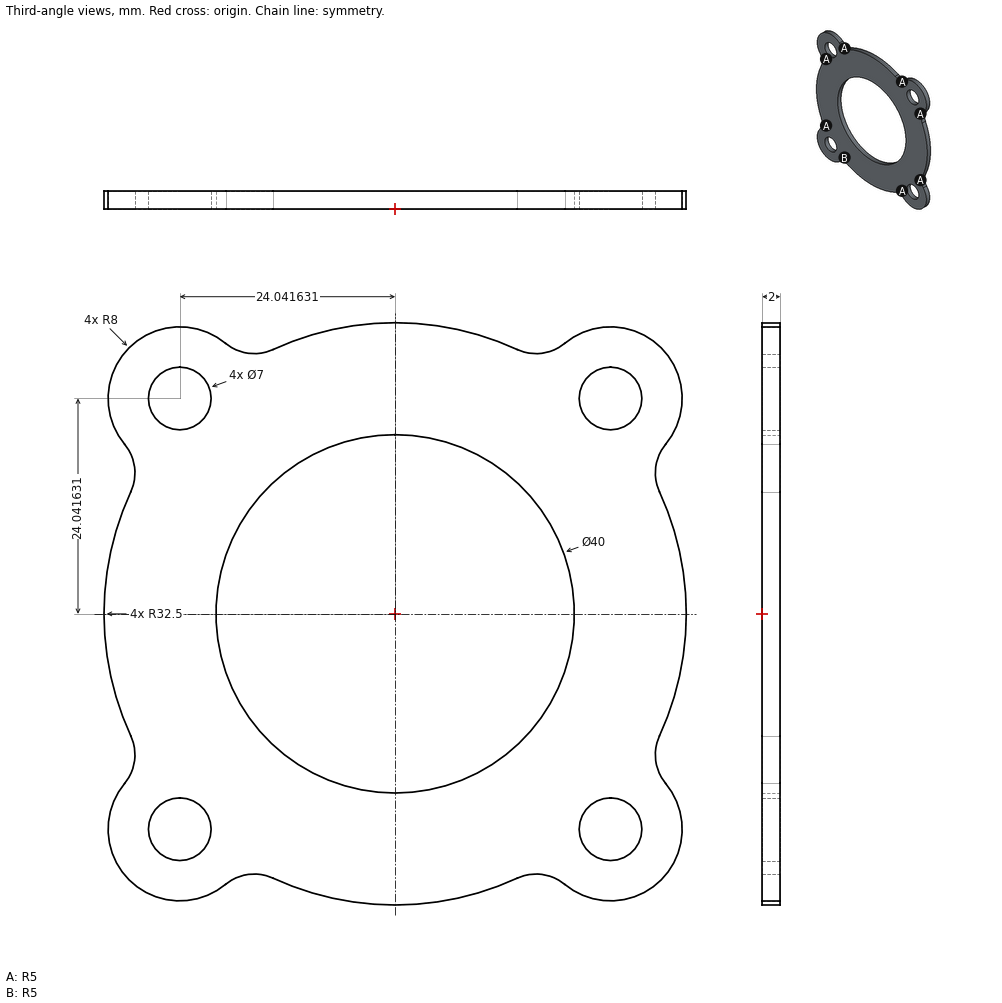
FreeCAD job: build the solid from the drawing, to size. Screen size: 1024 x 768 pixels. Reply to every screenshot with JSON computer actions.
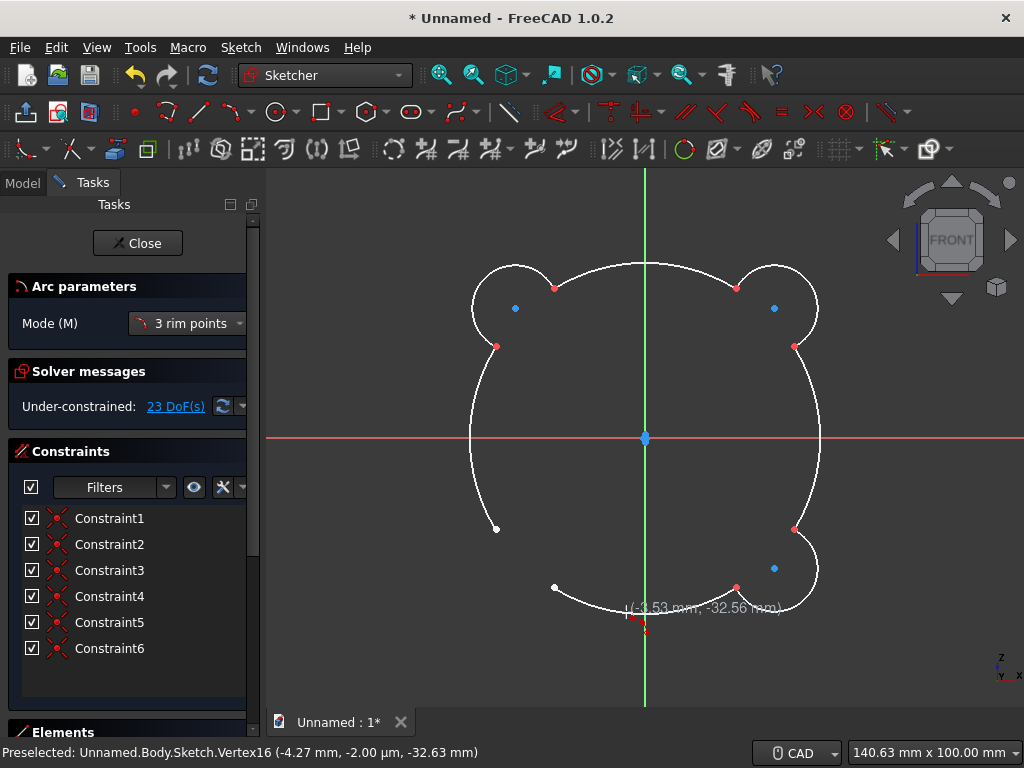
{"action": "left_click", "coordinate": [554, 588]}
{"action": "left_click", "coordinate": [496, 530]}
{"action": "left_click", "coordinate": [485, 598]}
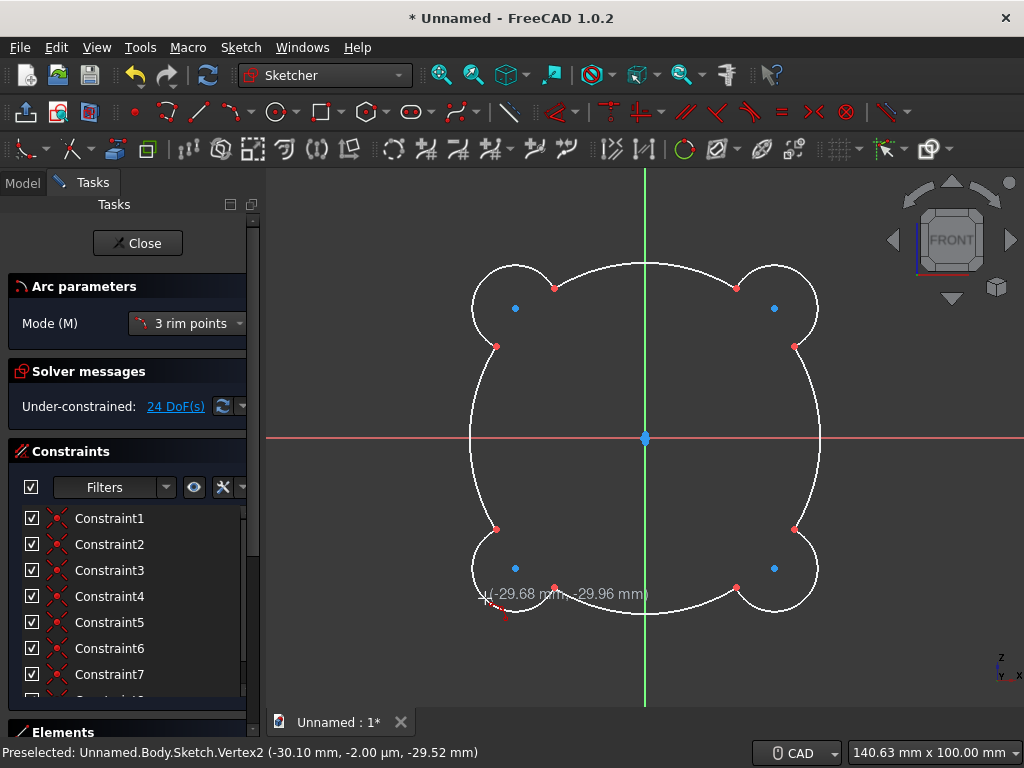
{"action": "left_click", "coordinate": [276, 112]}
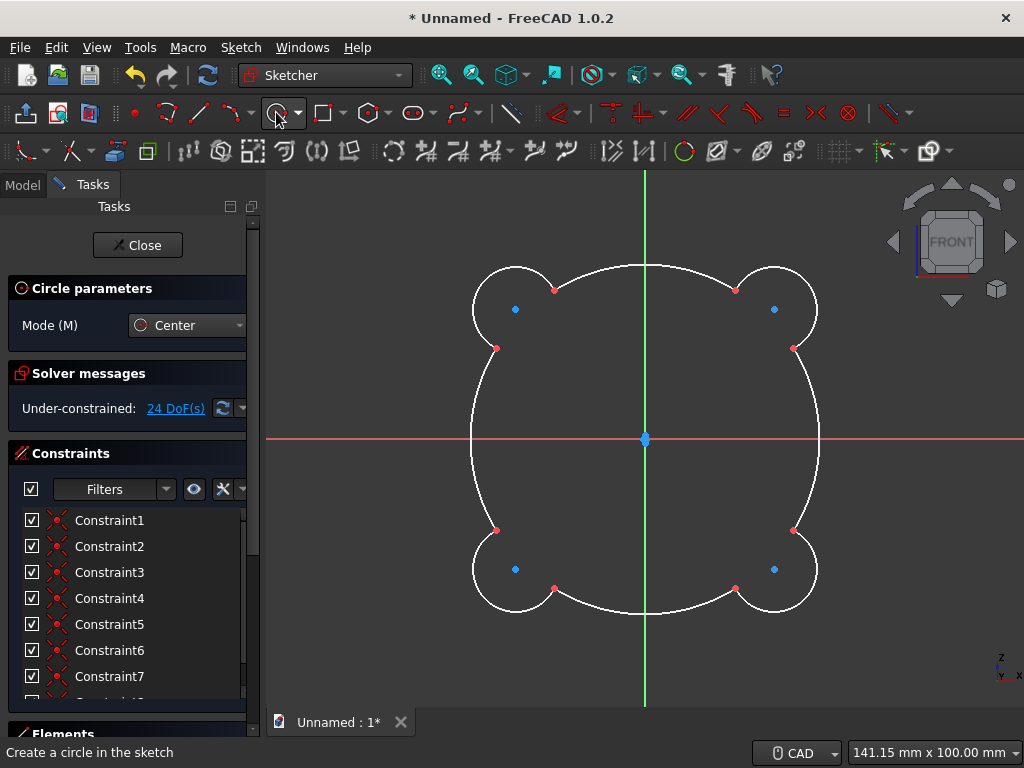
{"action": "left_click", "coordinate": [516, 309]}
{"action": "left_click", "coordinate": [529, 296]}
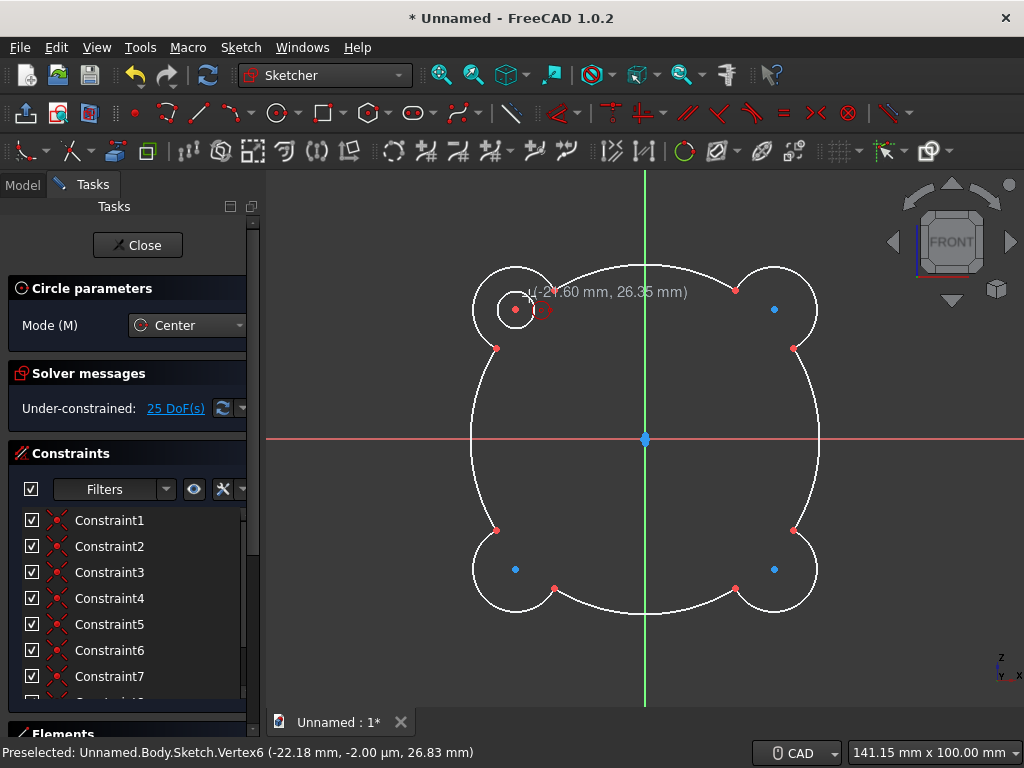
{"action": "left_click", "coordinate": [774, 309]}
{"action": "left_click", "coordinate": [787, 296]}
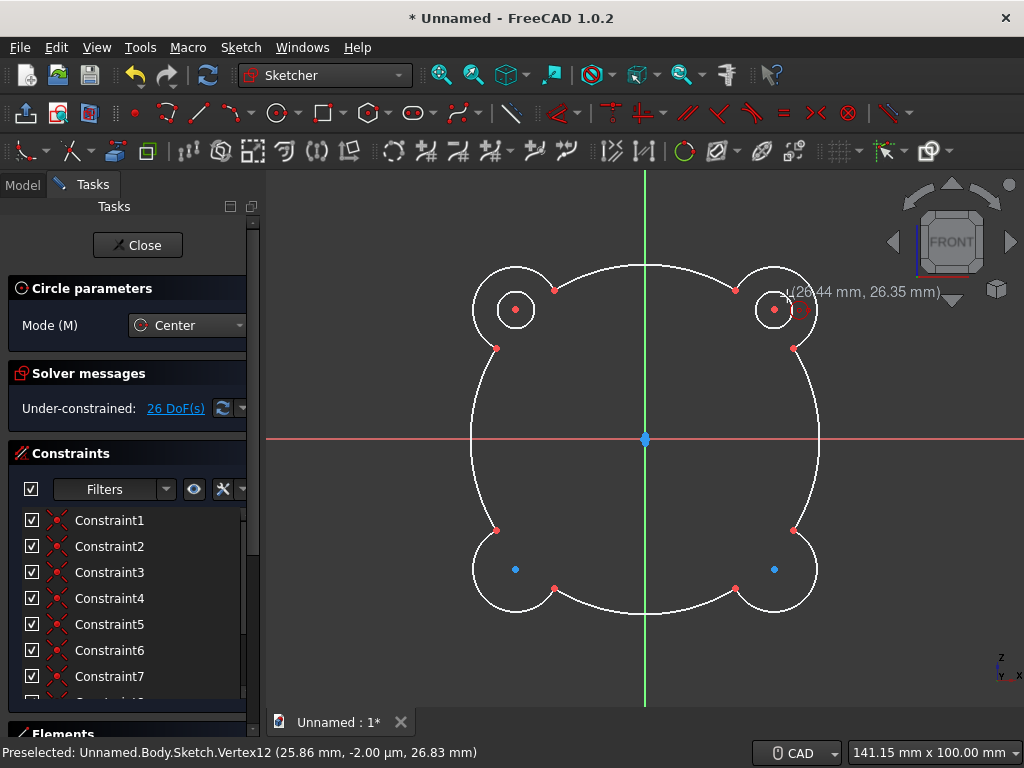
{"action": "left_click", "coordinate": [516, 568]}
{"action": "left_click", "coordinate": [529, 554]}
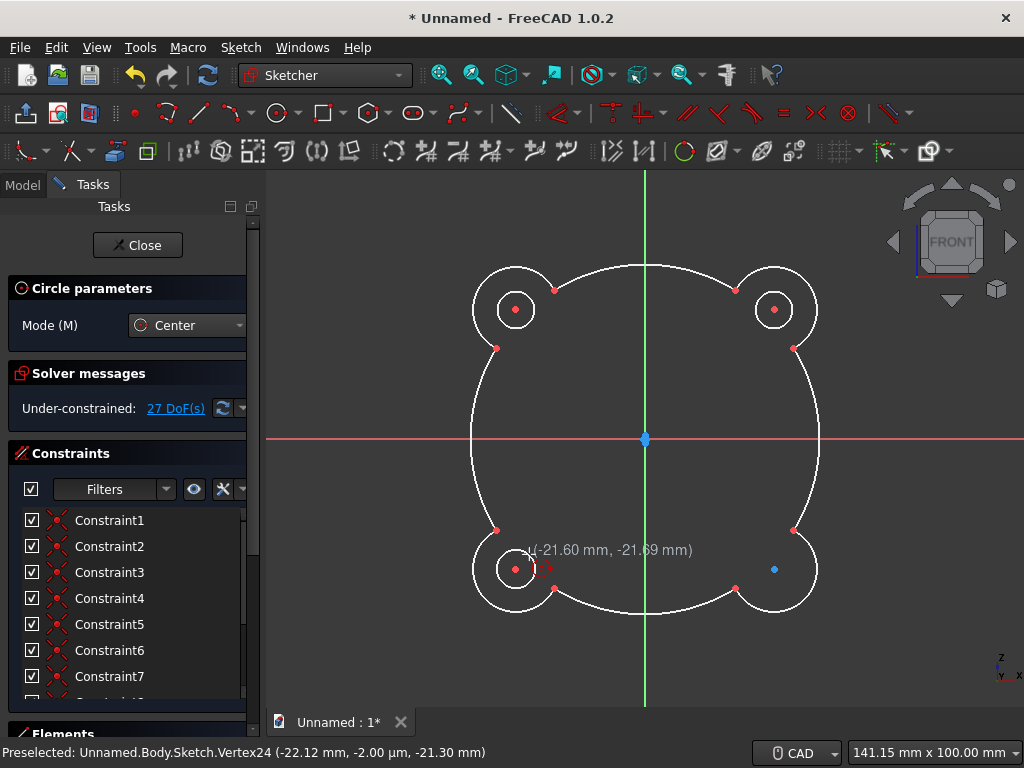
{"action": "left_click", "coordinate": [645, 438]}
{"action": "left_click", "coordinate": [721, 363]}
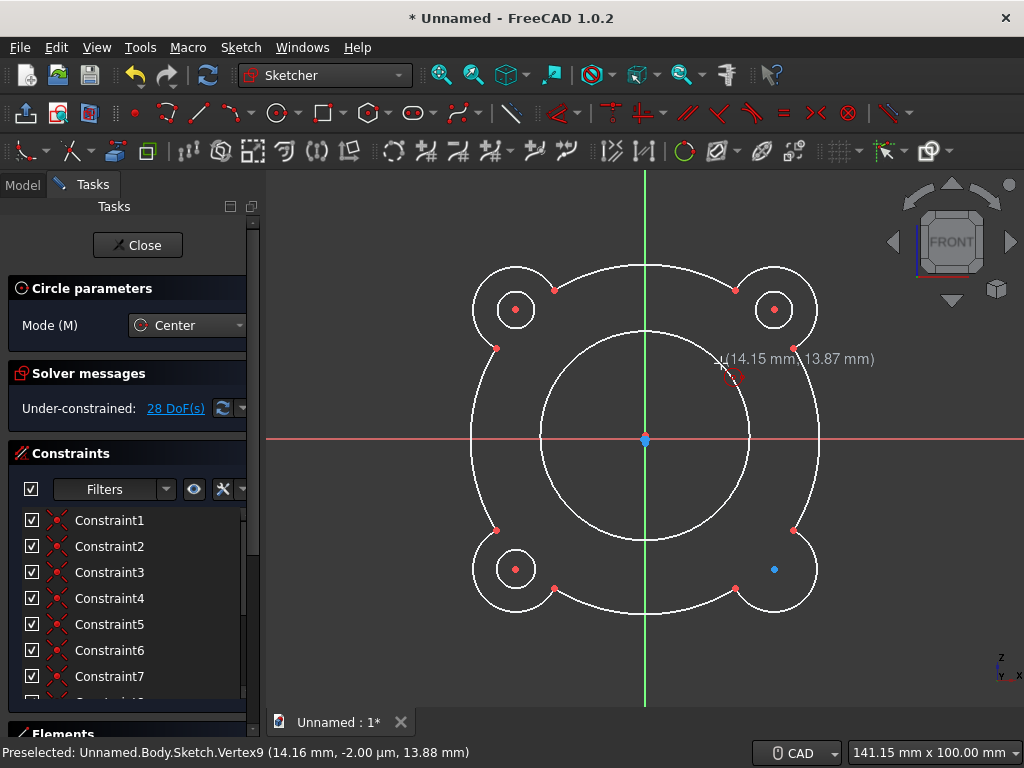
{"action": "left_click", "coordinate": [774, 568]}
{"action": "left_click", "coordinate": [787, 554]}
{"action": "key", "text": "Escape"}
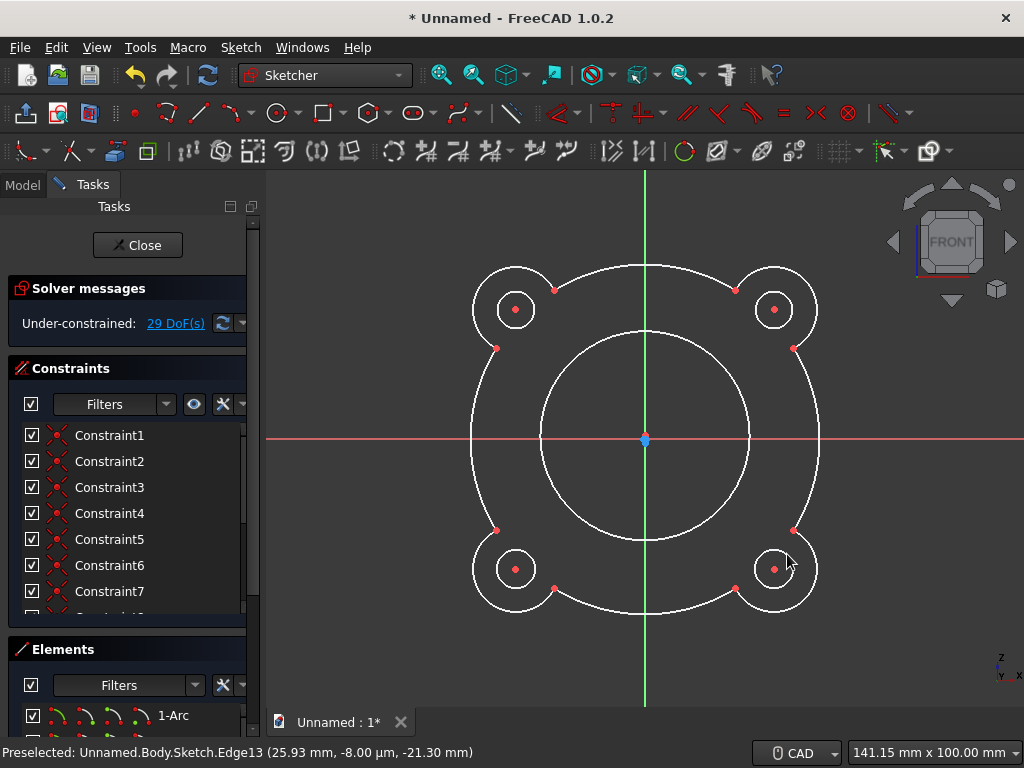
{"action": "left_click", "coordinate": [719, 362]}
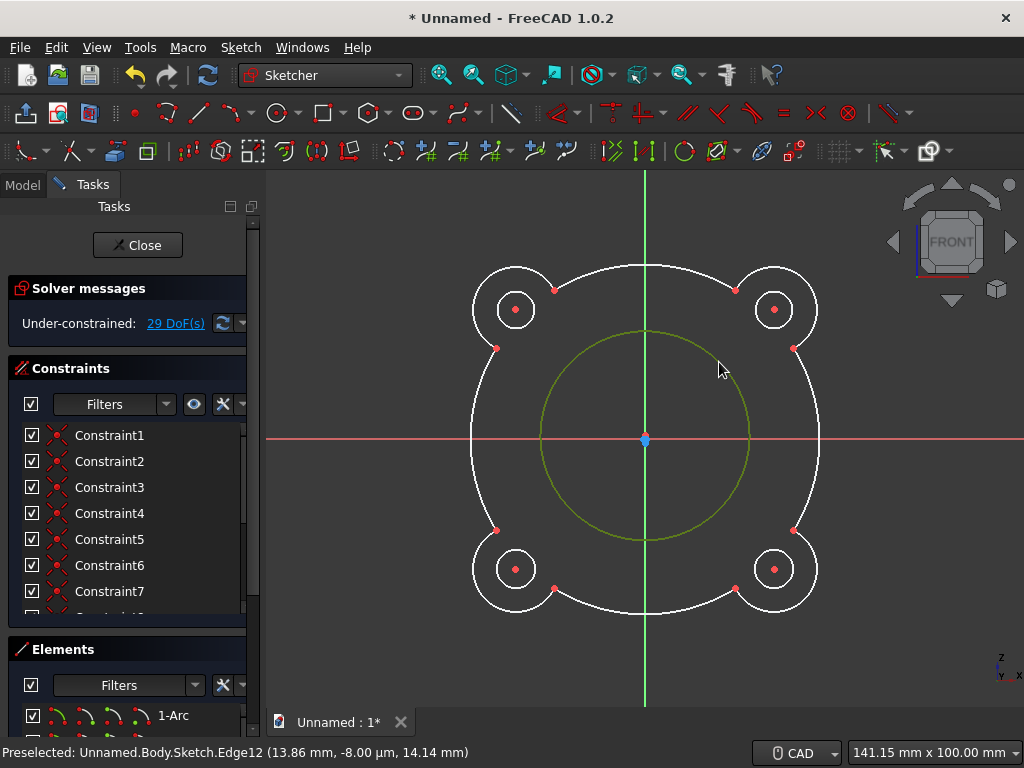
{"action": "left_click", "coordinate": [475, 401]}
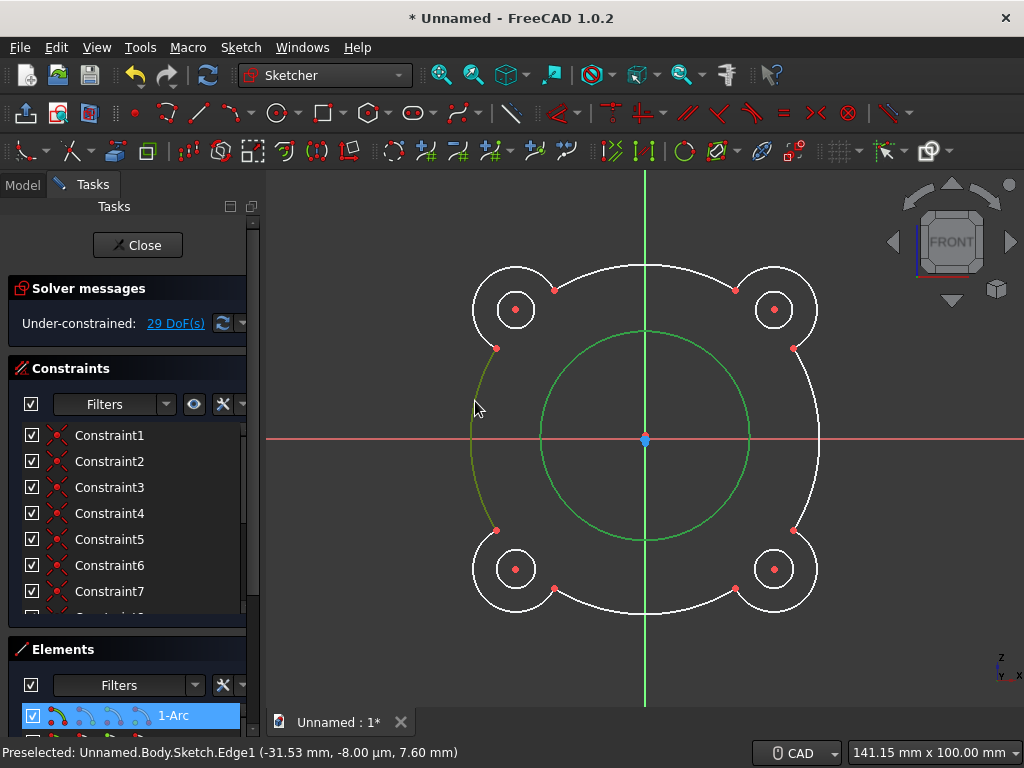
{"action": "left_click", "coordinate": [612, 114]}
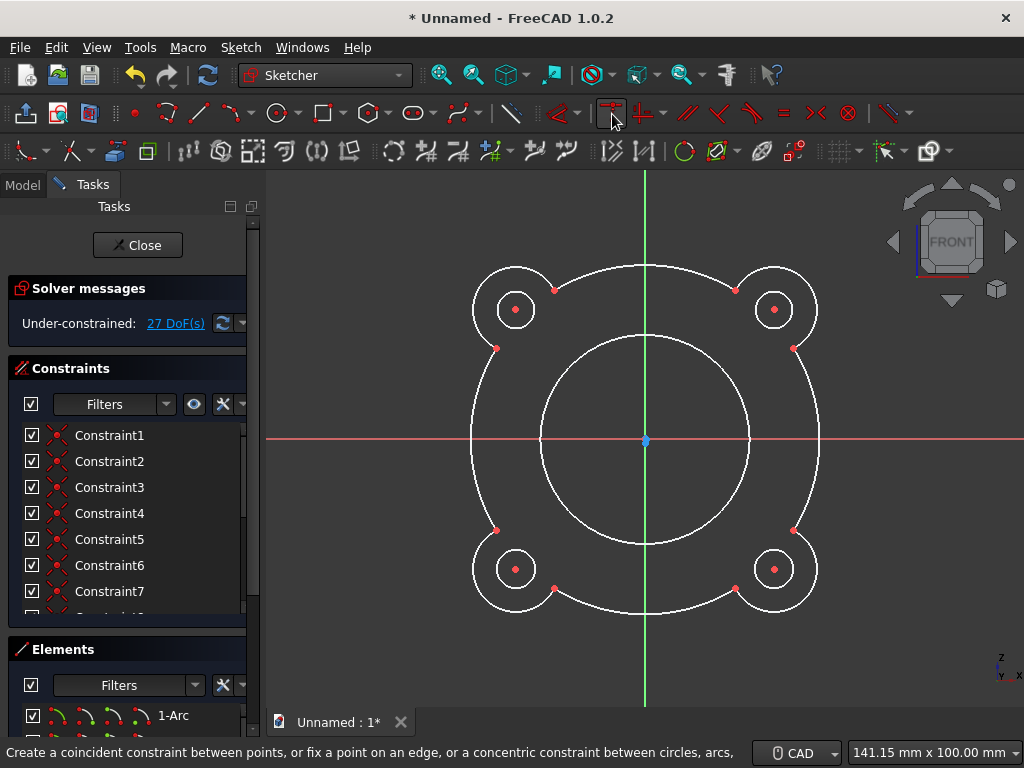
{"action": "left_click", "coordinate": [719, 365]}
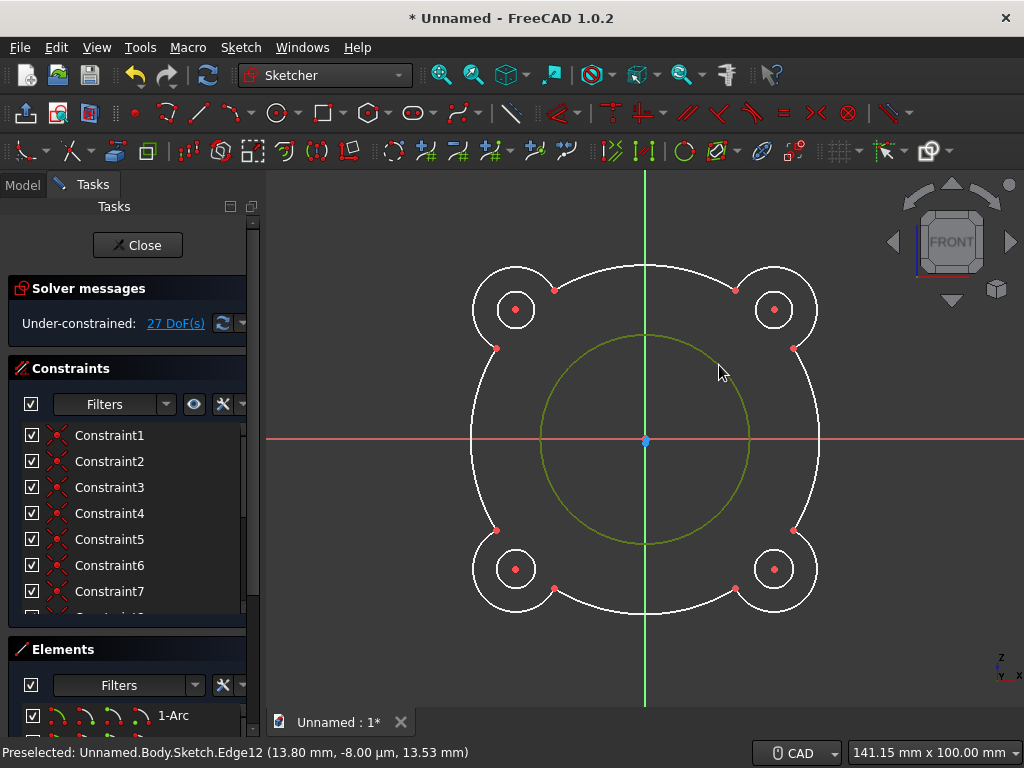
{"action": "left_click", "coordinate": [815, 478]}